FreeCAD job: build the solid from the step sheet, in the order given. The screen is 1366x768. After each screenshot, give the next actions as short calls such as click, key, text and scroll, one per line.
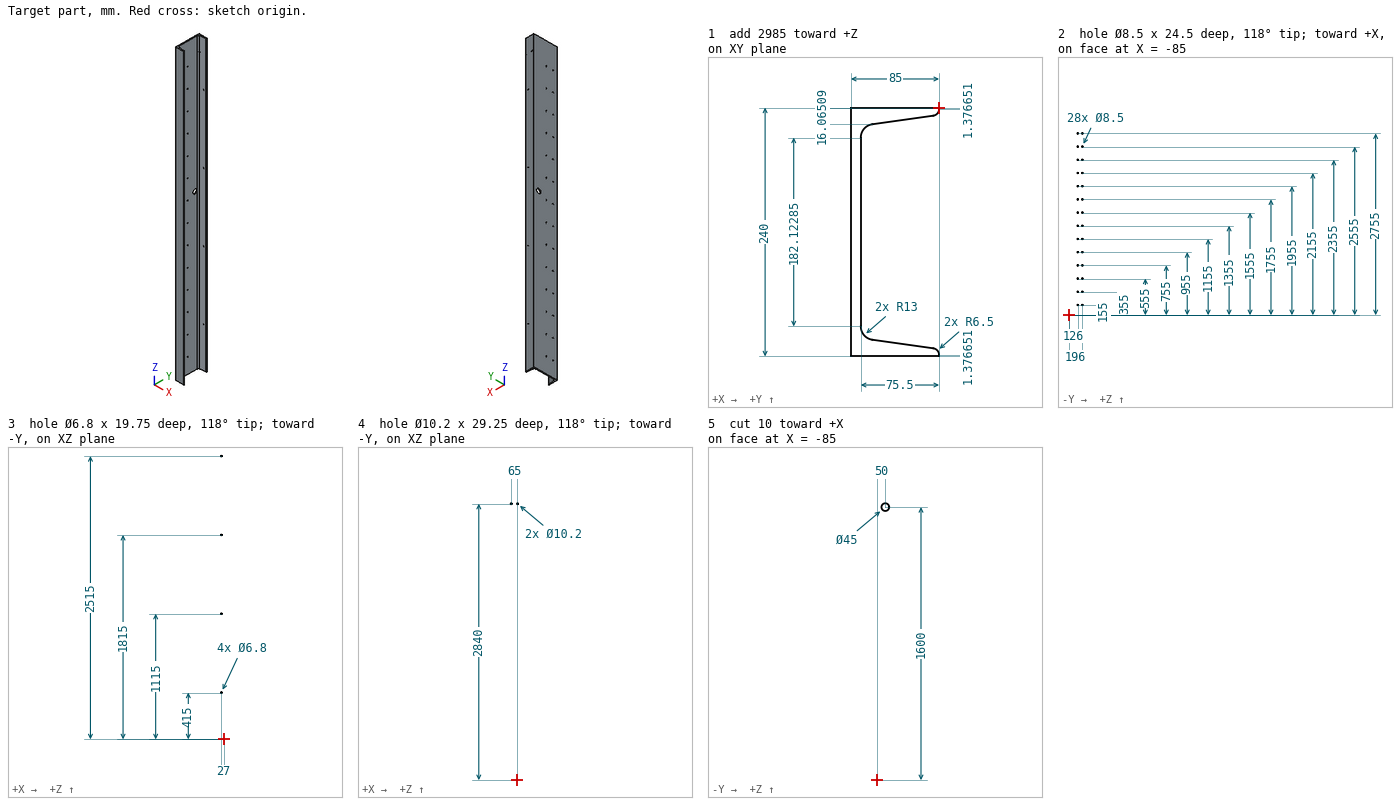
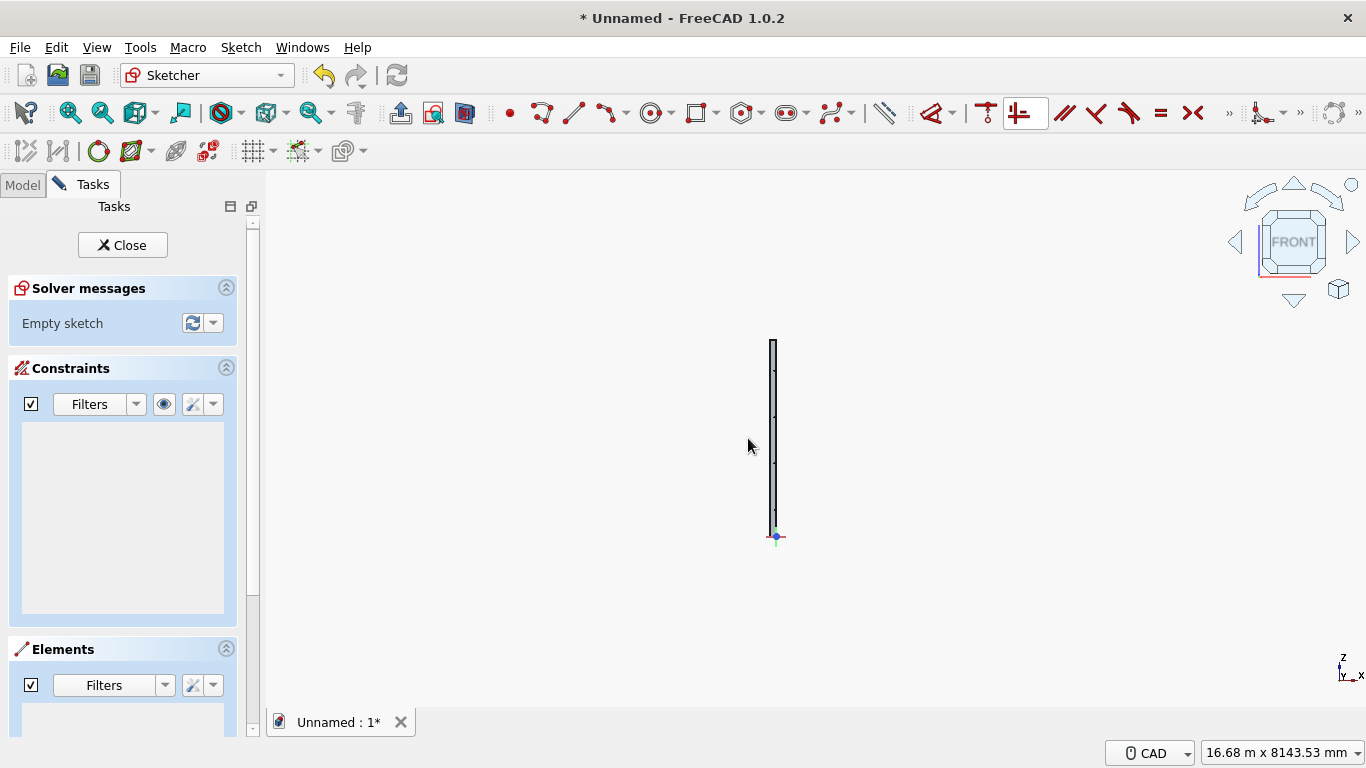
scroll(775, 345, up, 15)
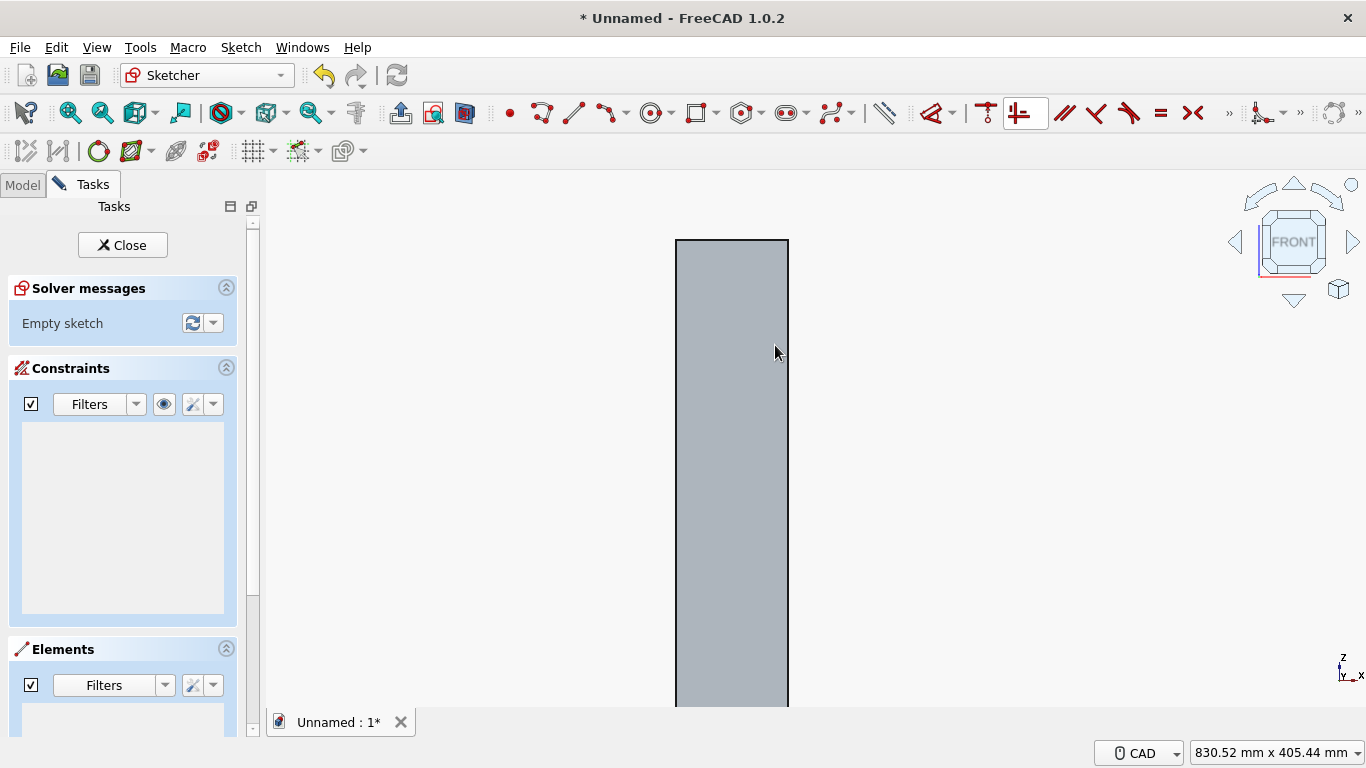
scroll(745, 431, up, 9)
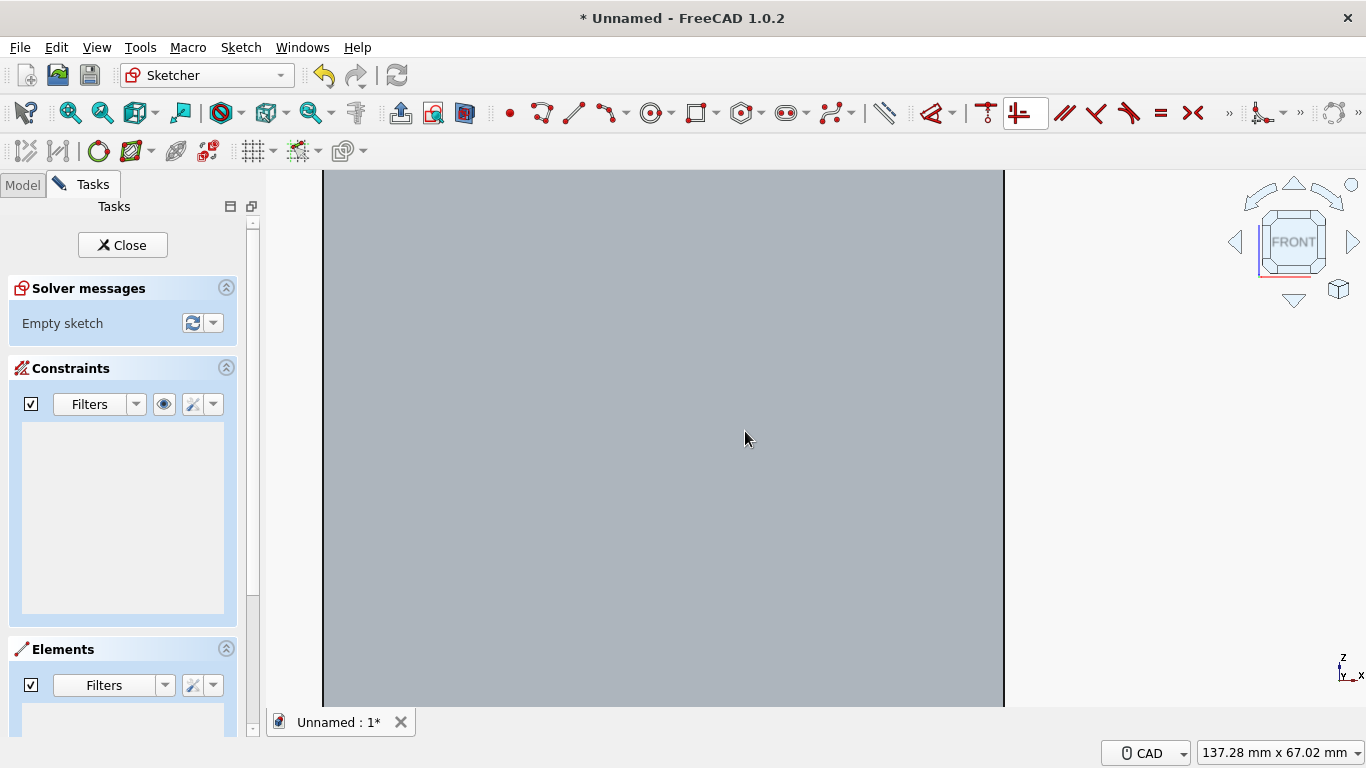
click(652, 114)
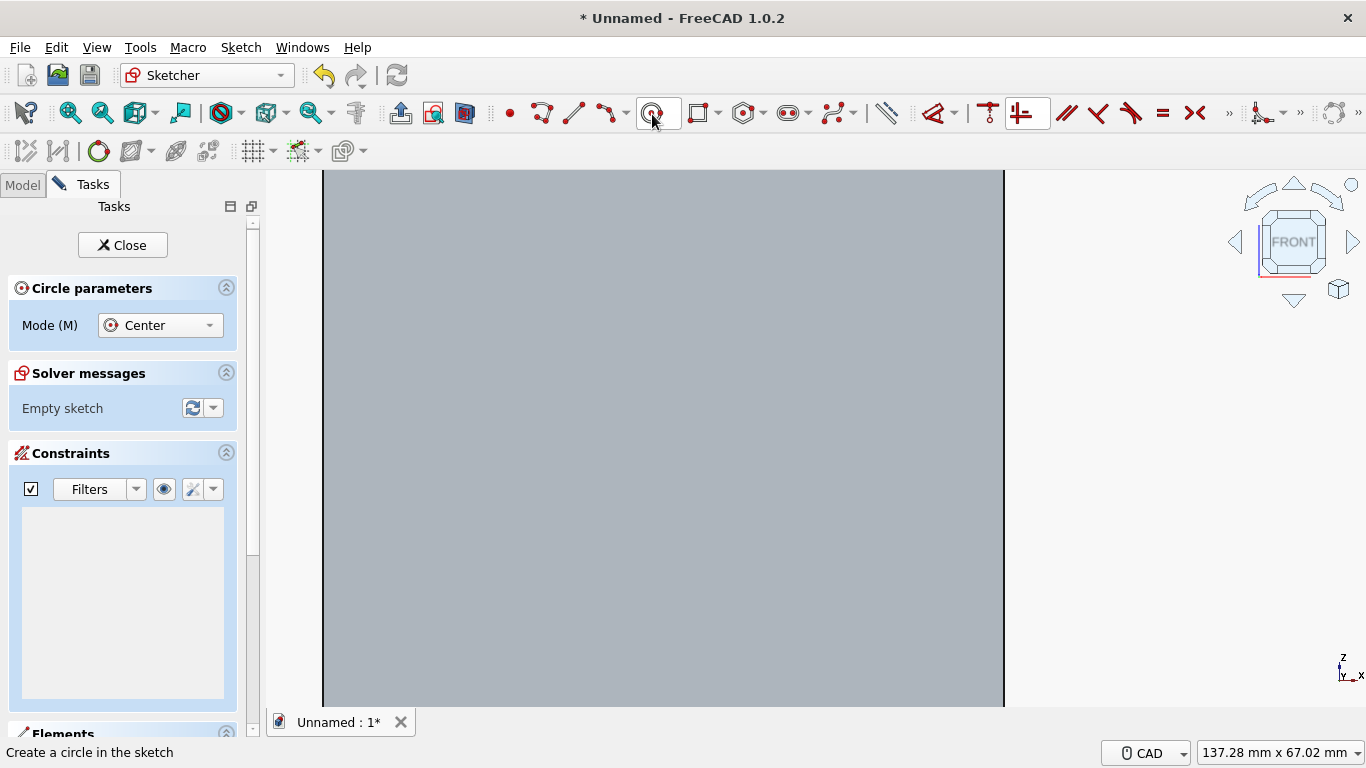
click(483, 435)
move(512, 406)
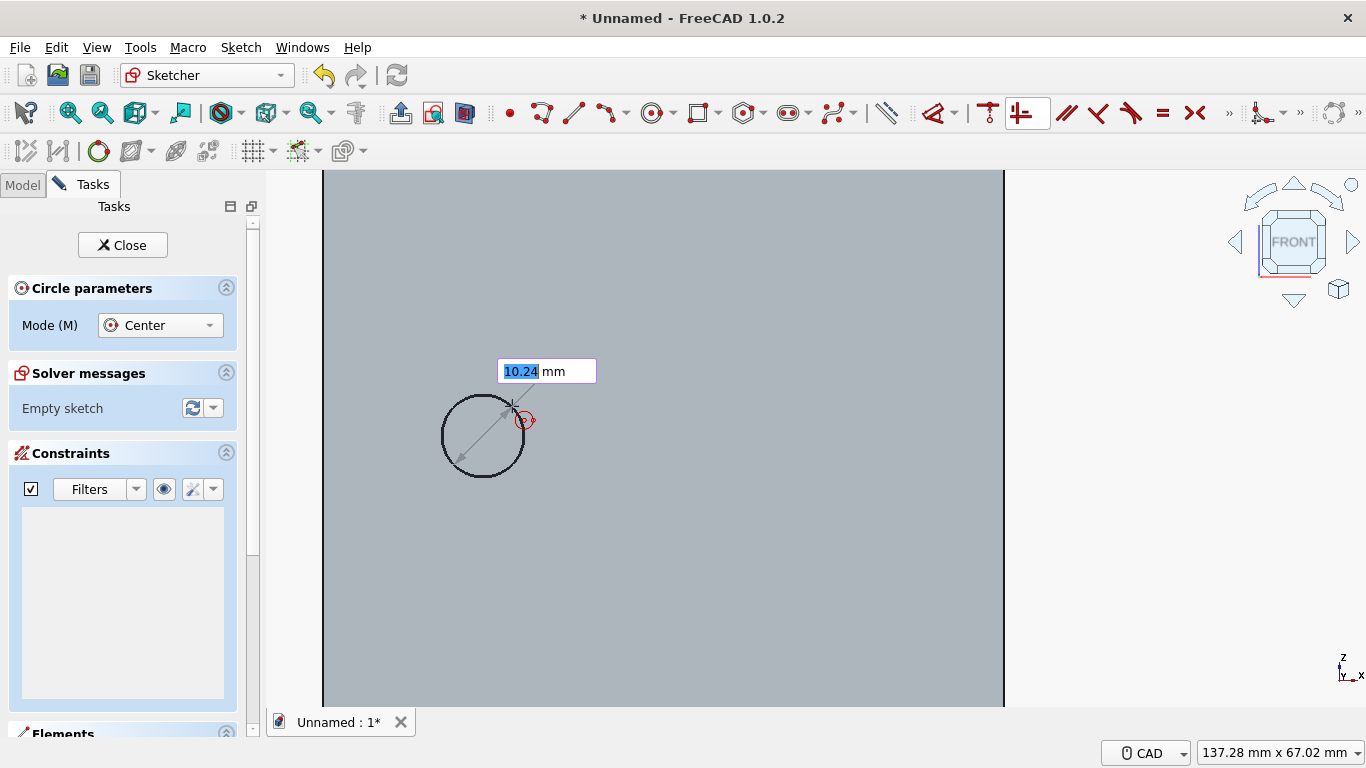
text(10.2)
key(Return)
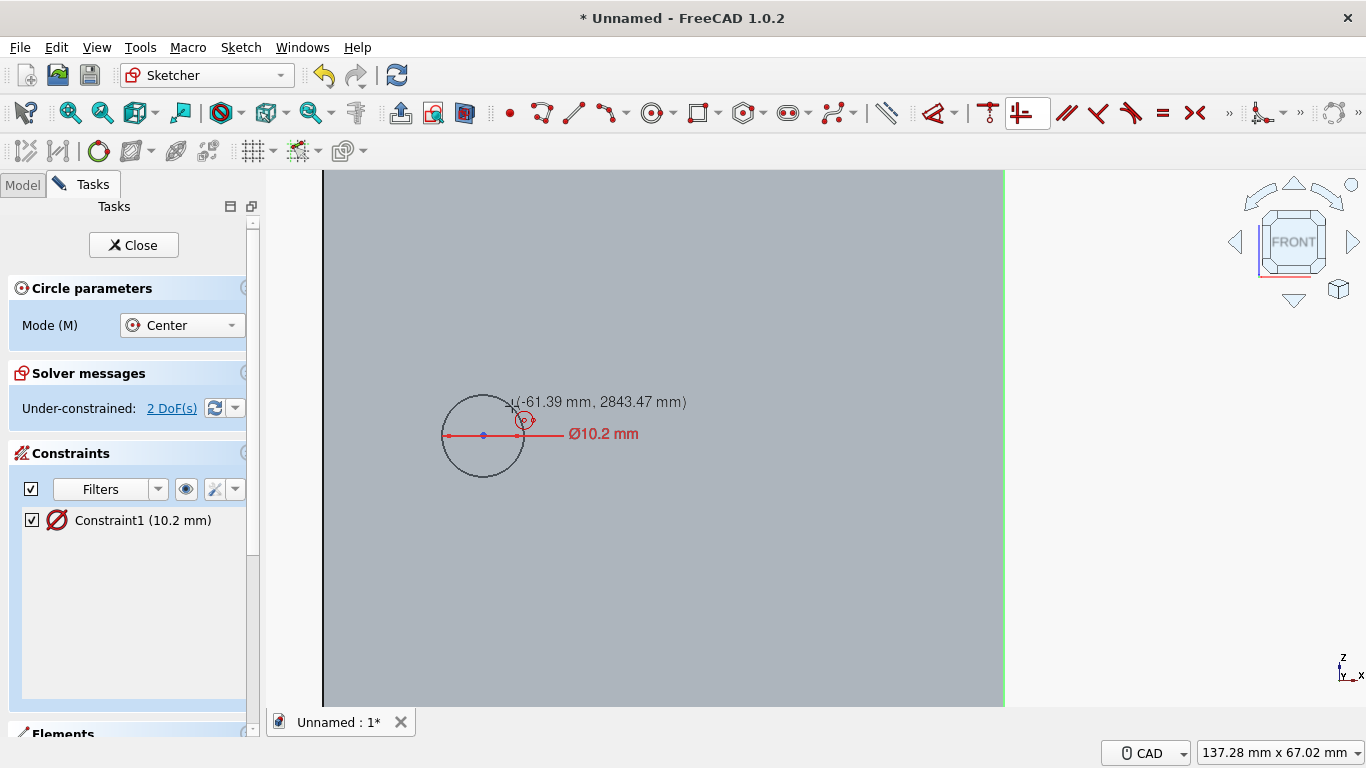
click(1004, 435)
move(1033, 406)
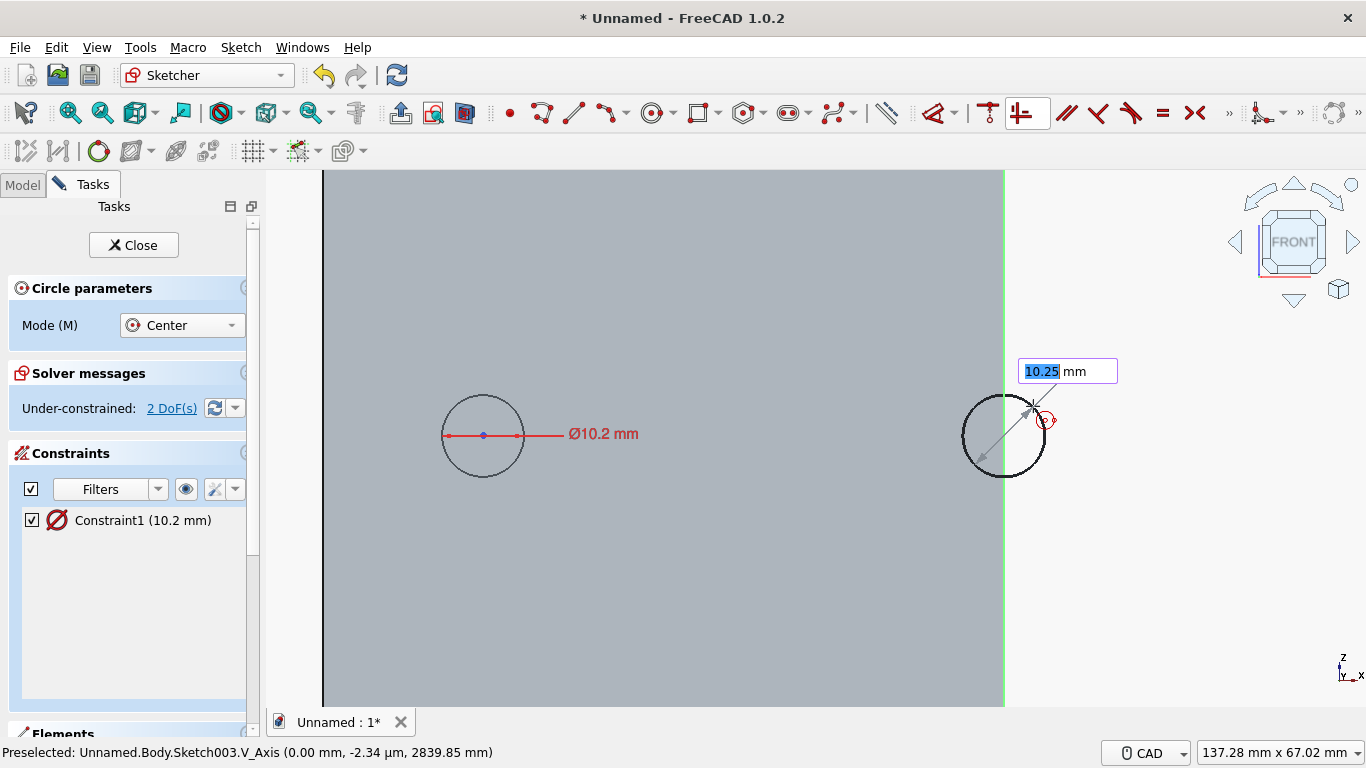
text(10.2)
key(Return)
key(Escape)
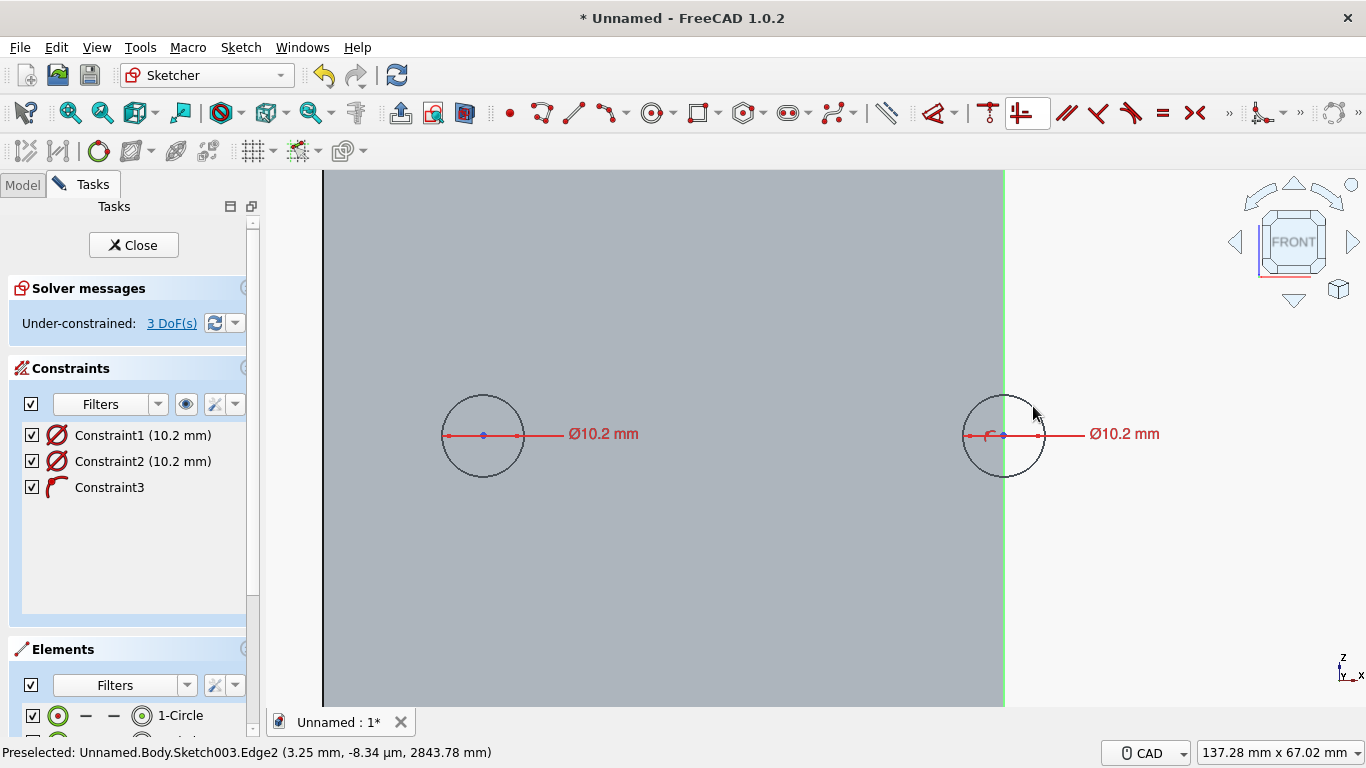
click(483, 436)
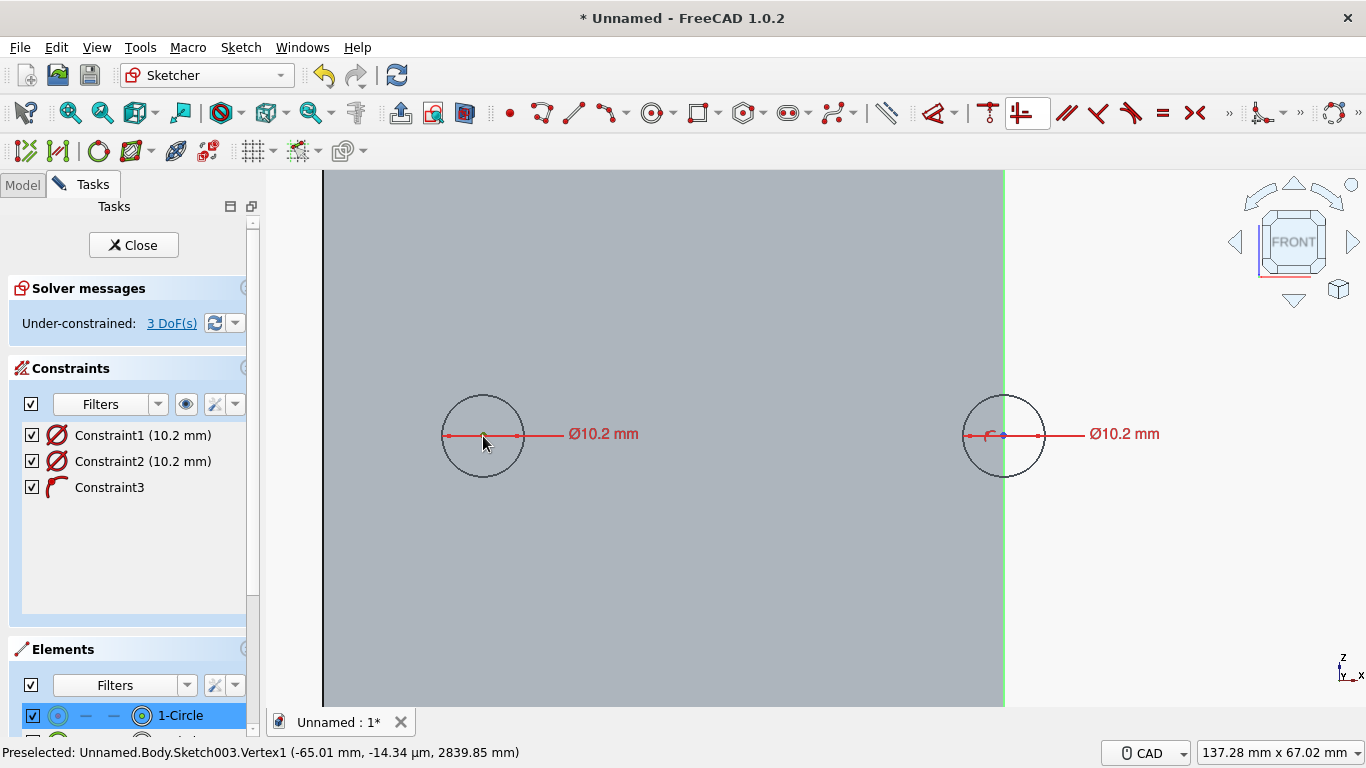
click(1004, 436)